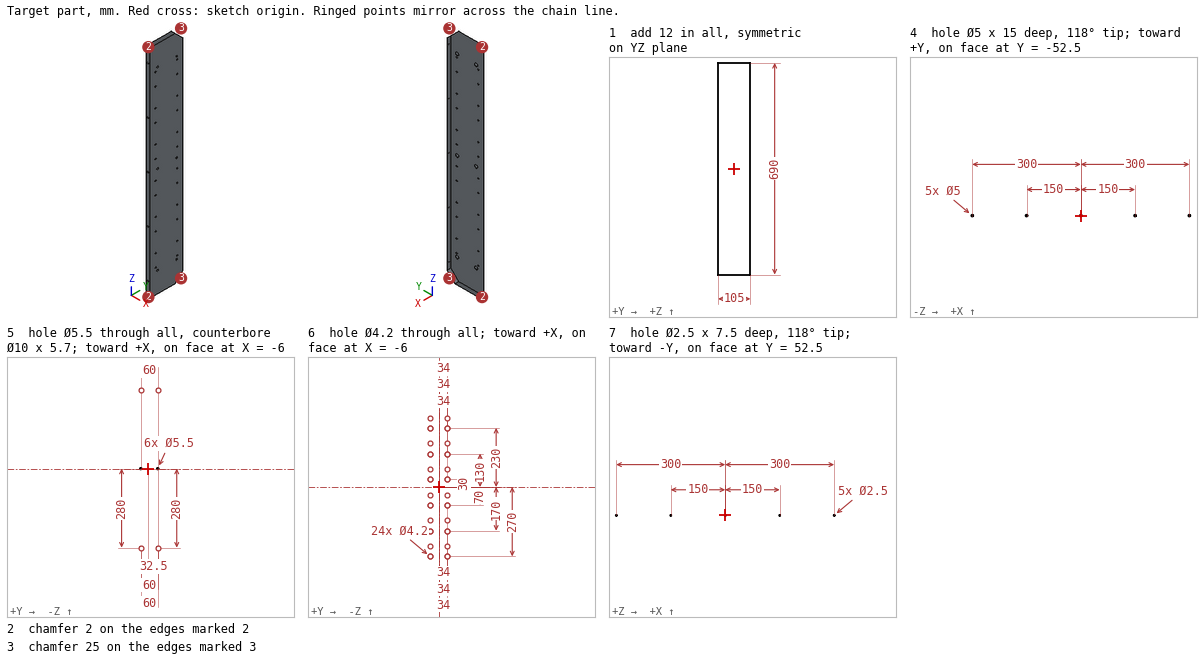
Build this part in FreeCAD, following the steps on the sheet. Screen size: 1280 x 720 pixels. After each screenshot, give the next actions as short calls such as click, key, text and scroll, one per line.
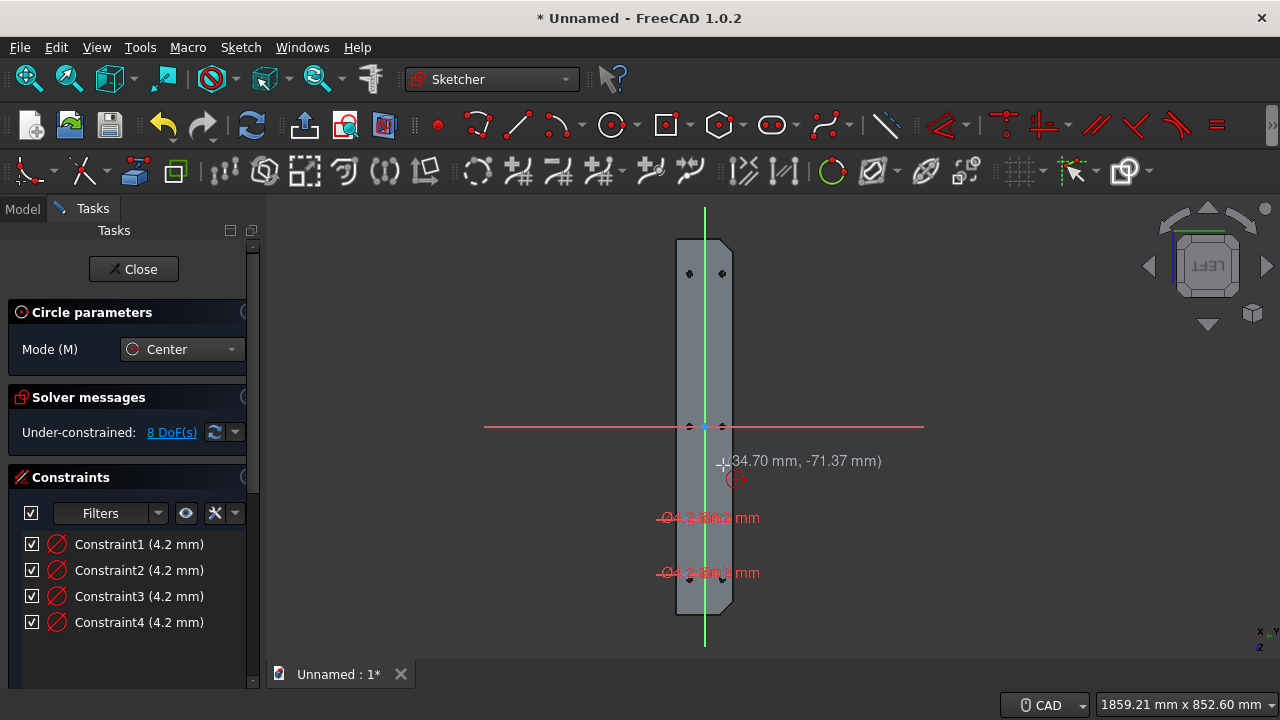
click(723, 465)
move(724, 464)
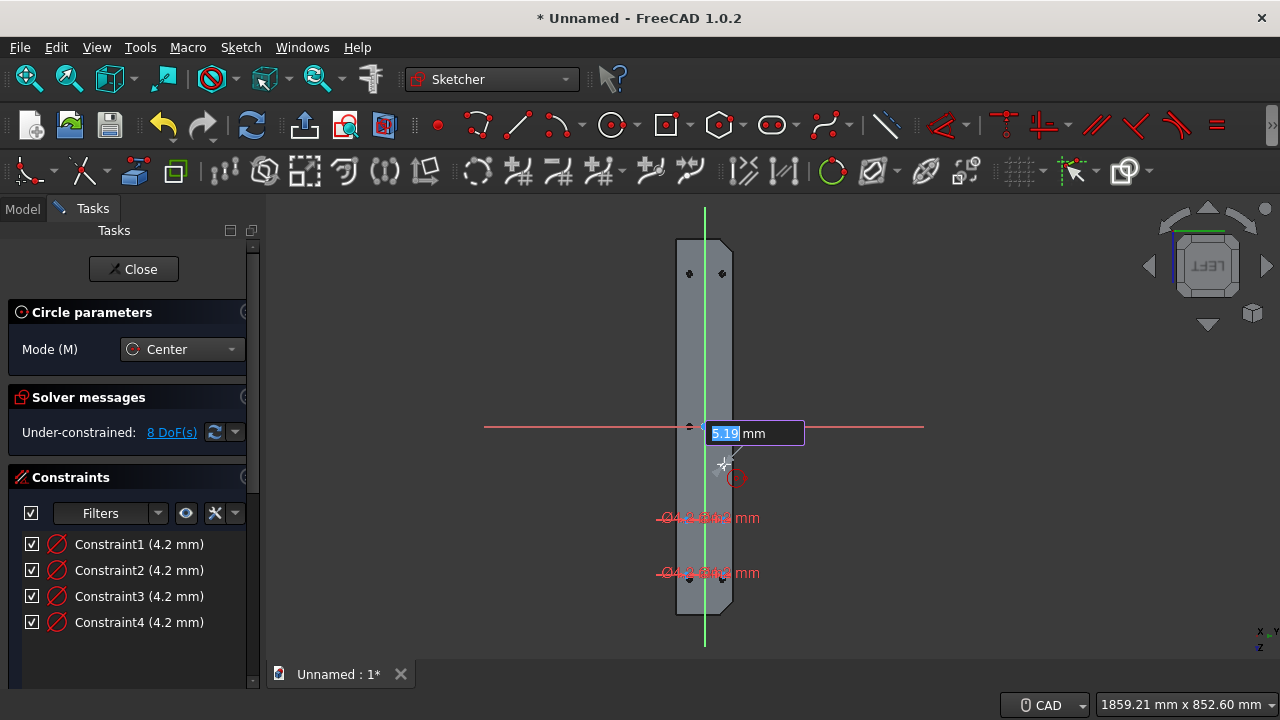
text(4.2)
key(Return)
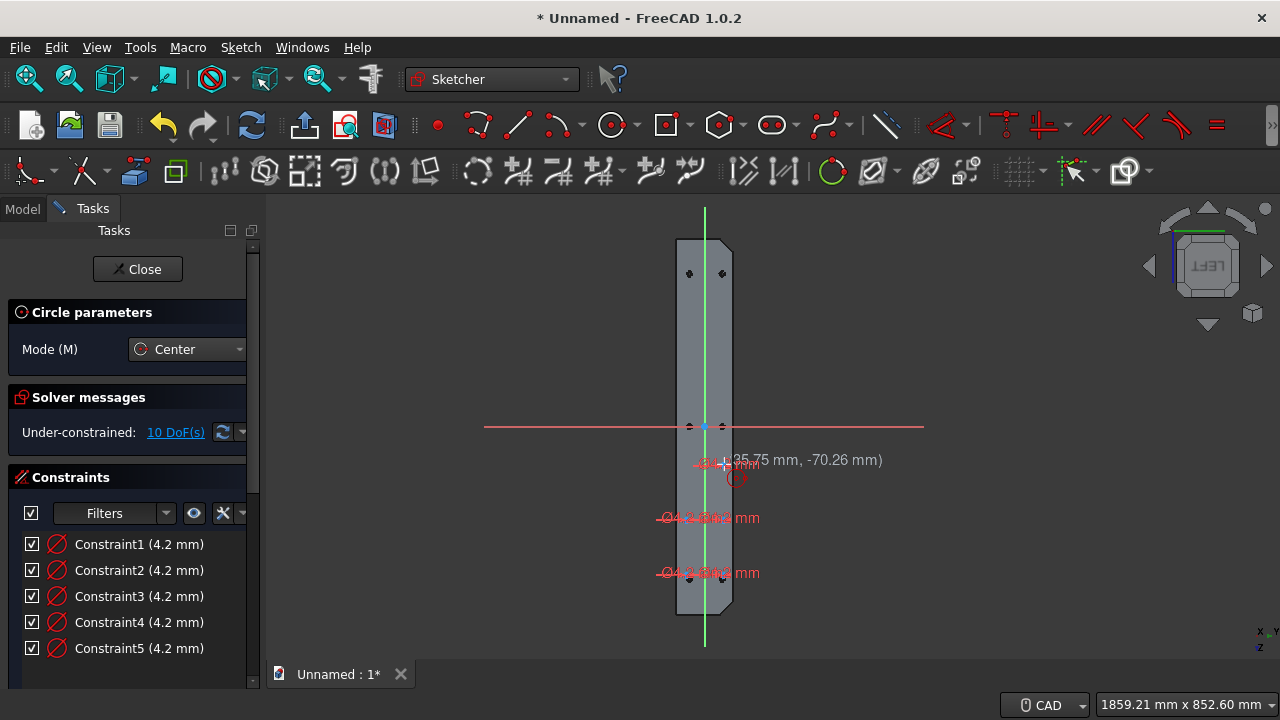
scroll(686, 465, up, 15)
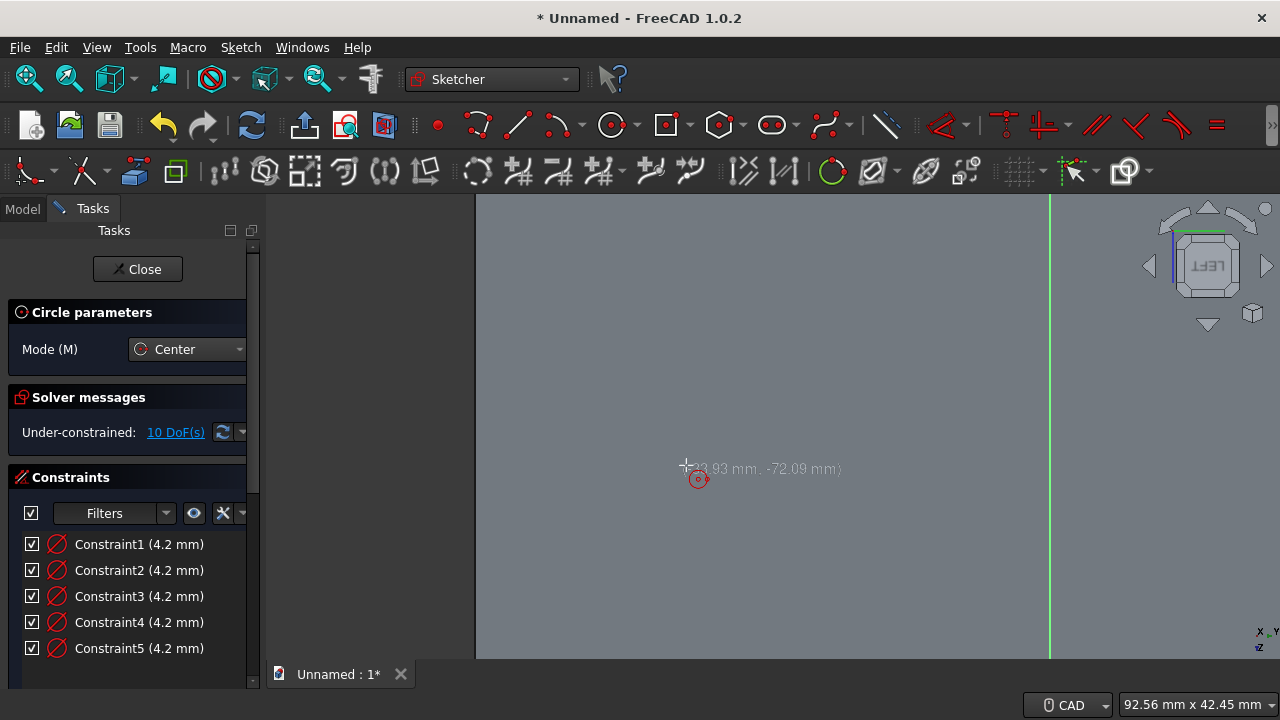
scroll(686, 465, down, 15)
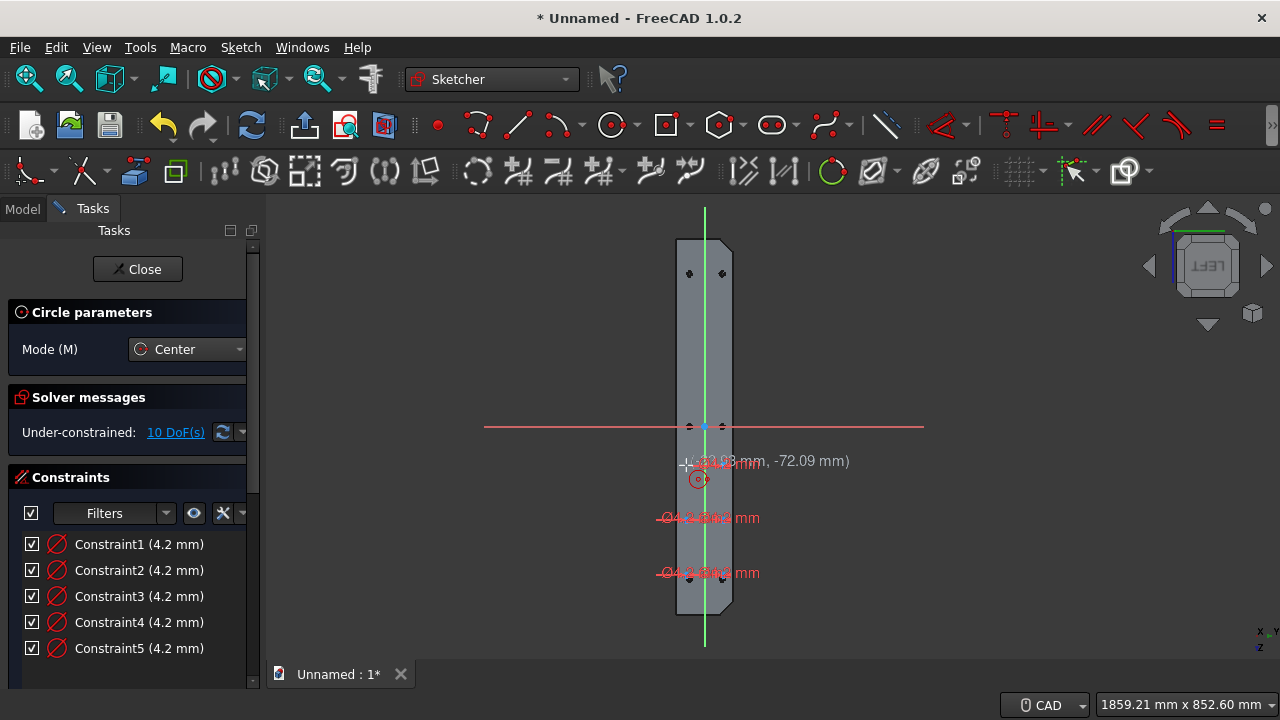
click(686, 465)
move(687, 464)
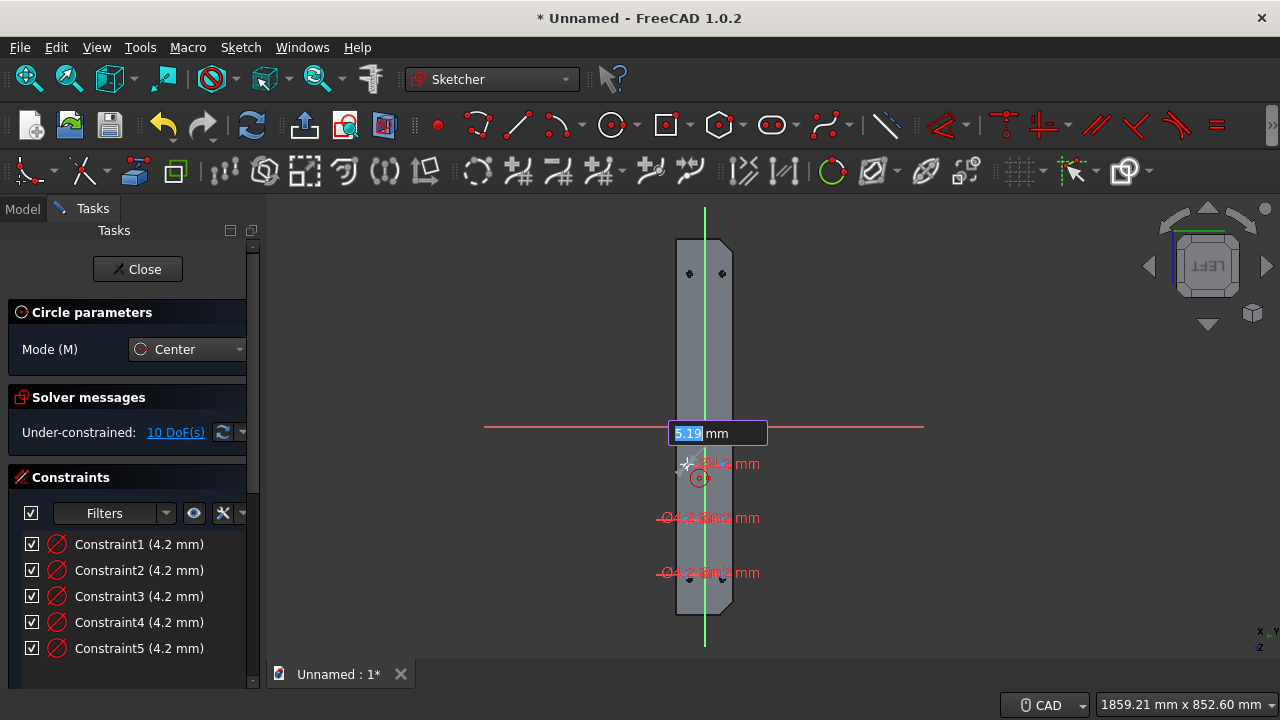
text(4.2)
key(Return)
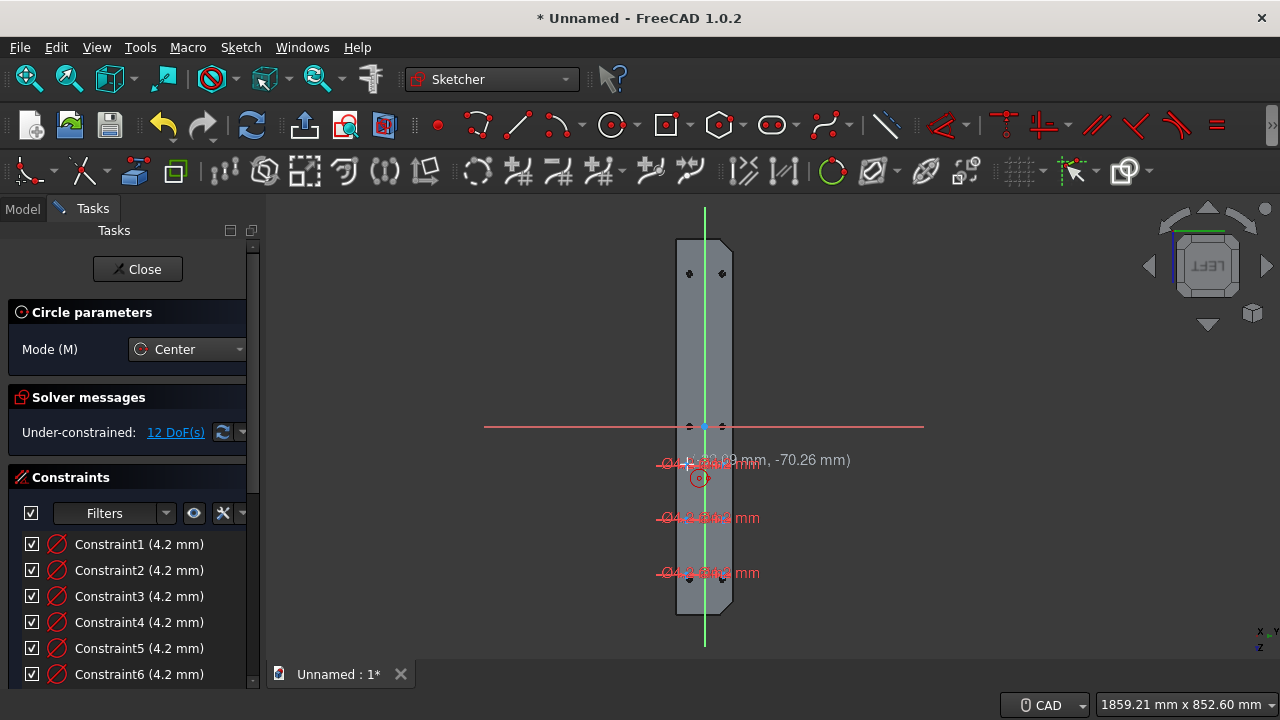
scroll(723, 410, up, 15)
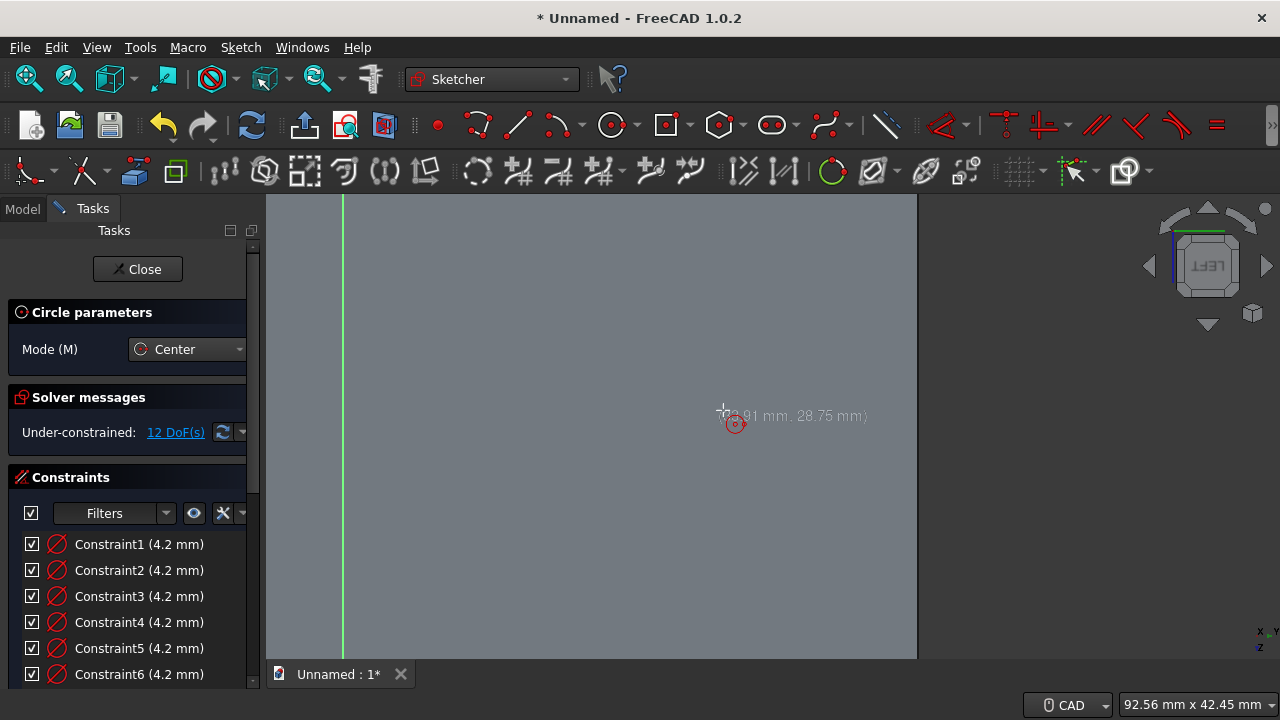
scroll(723, 410, down, 15)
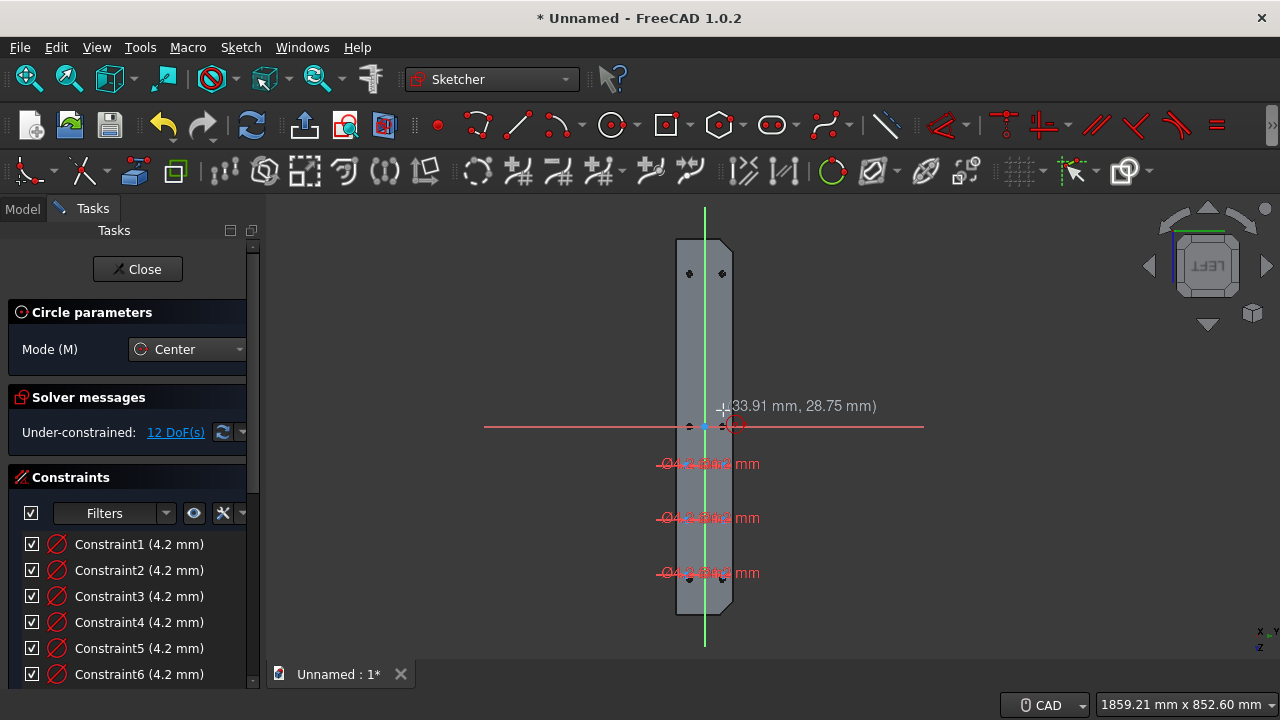
click(723, 410)
move(724, 410)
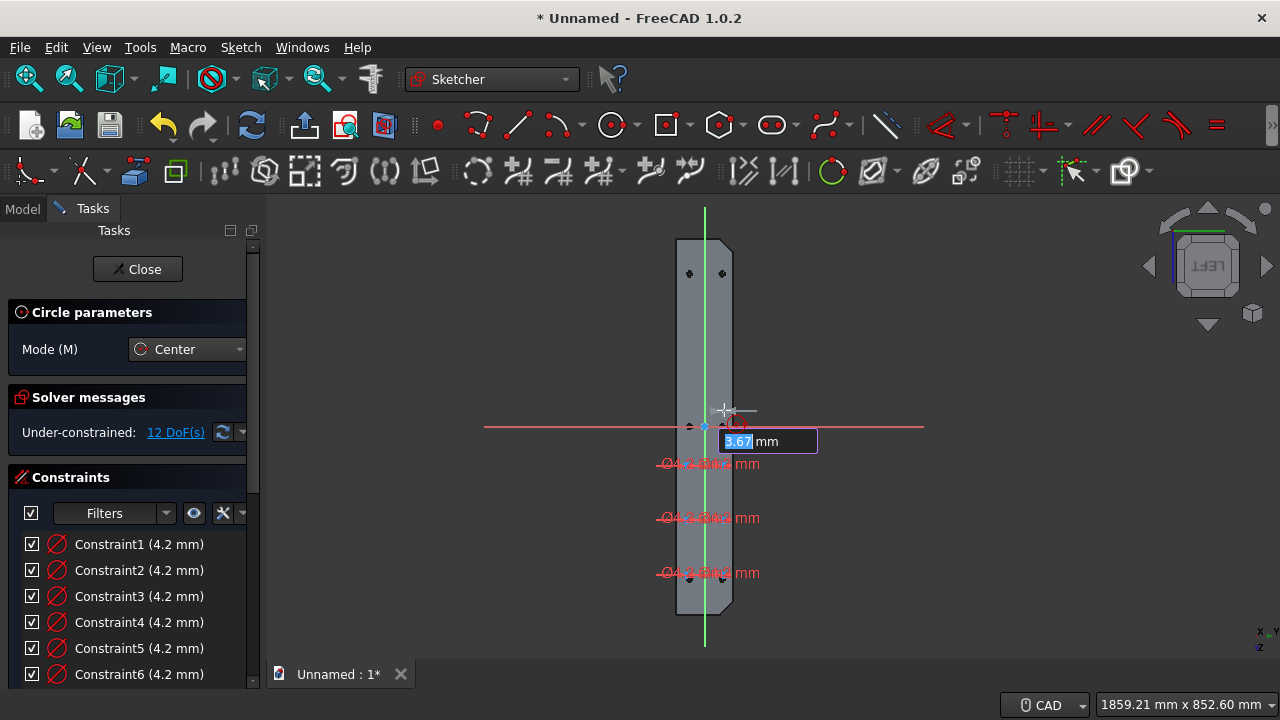
text(4.2)
key(Return)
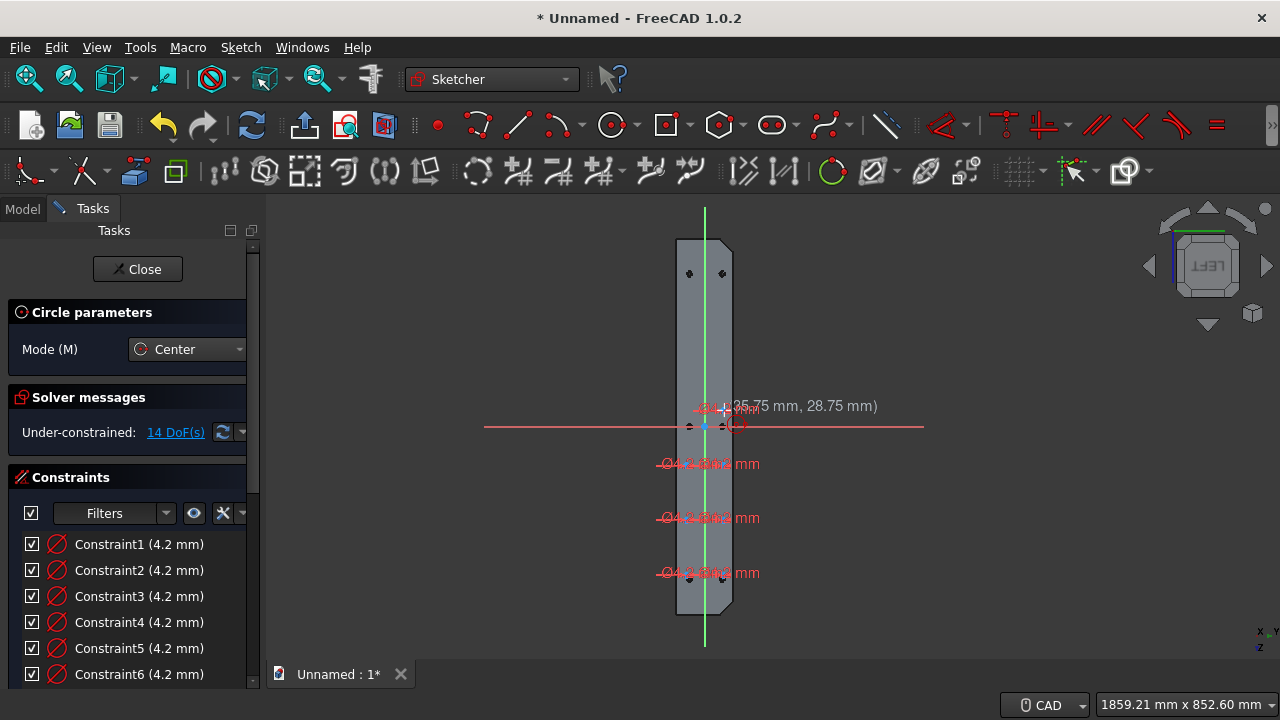
scroll(686, 410, up, 15)